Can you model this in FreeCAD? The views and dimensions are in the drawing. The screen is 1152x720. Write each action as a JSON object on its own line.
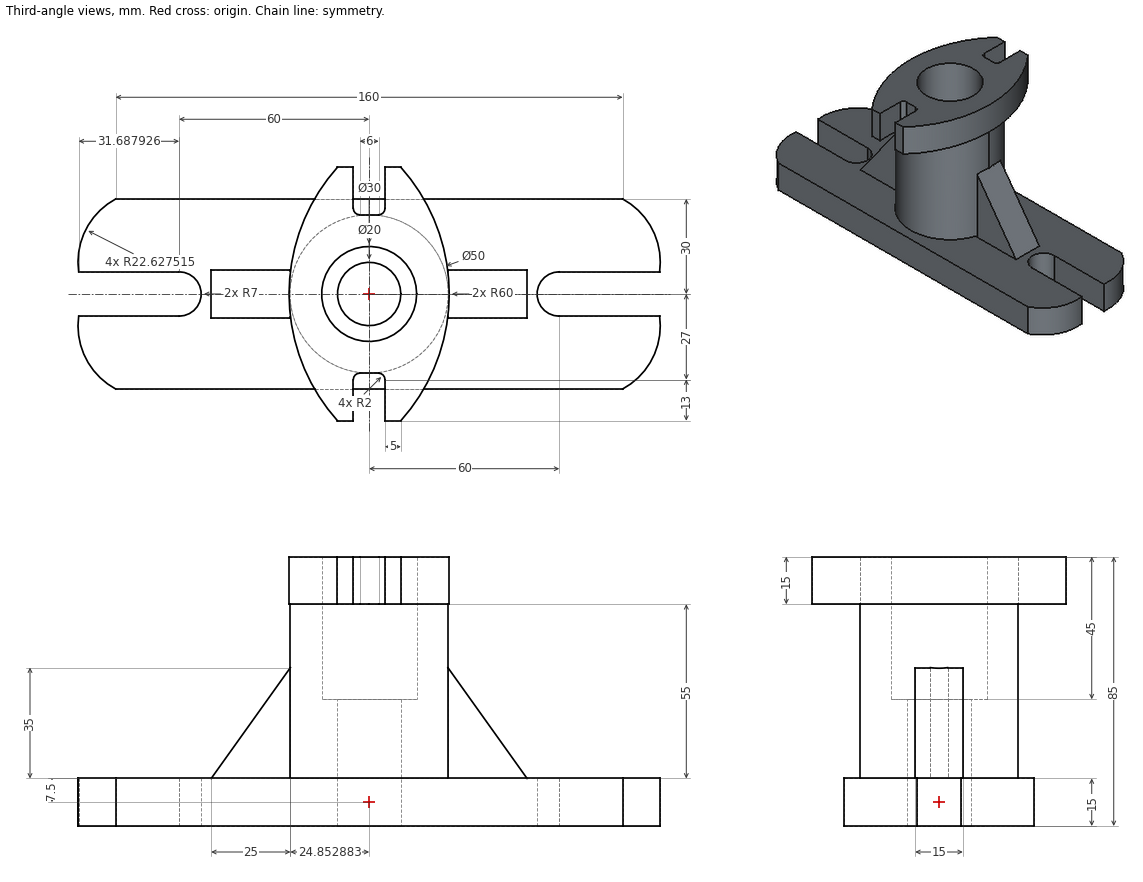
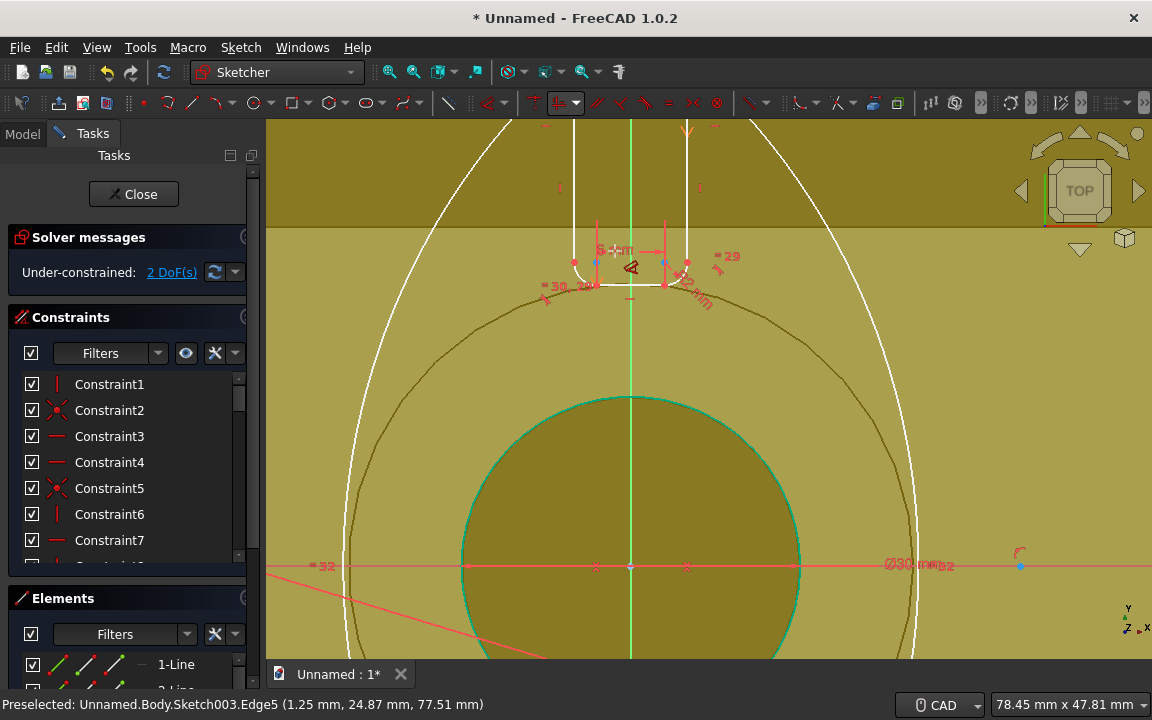
{"action": "scroll", "coordinate": [646, 286], "scroll_direction": "down", "scroll_amount": 5}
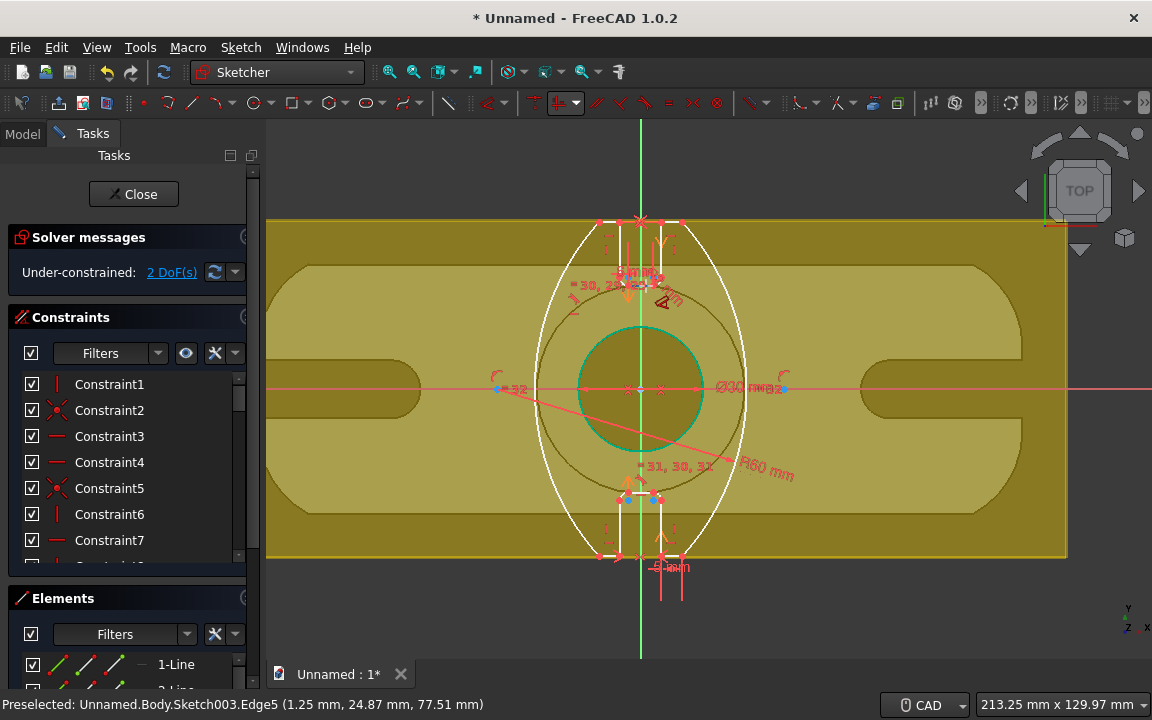
{"action": "left_click", "coordinate": [661, 518]}
{"action": "left_click", "coordinate": [695, 516]}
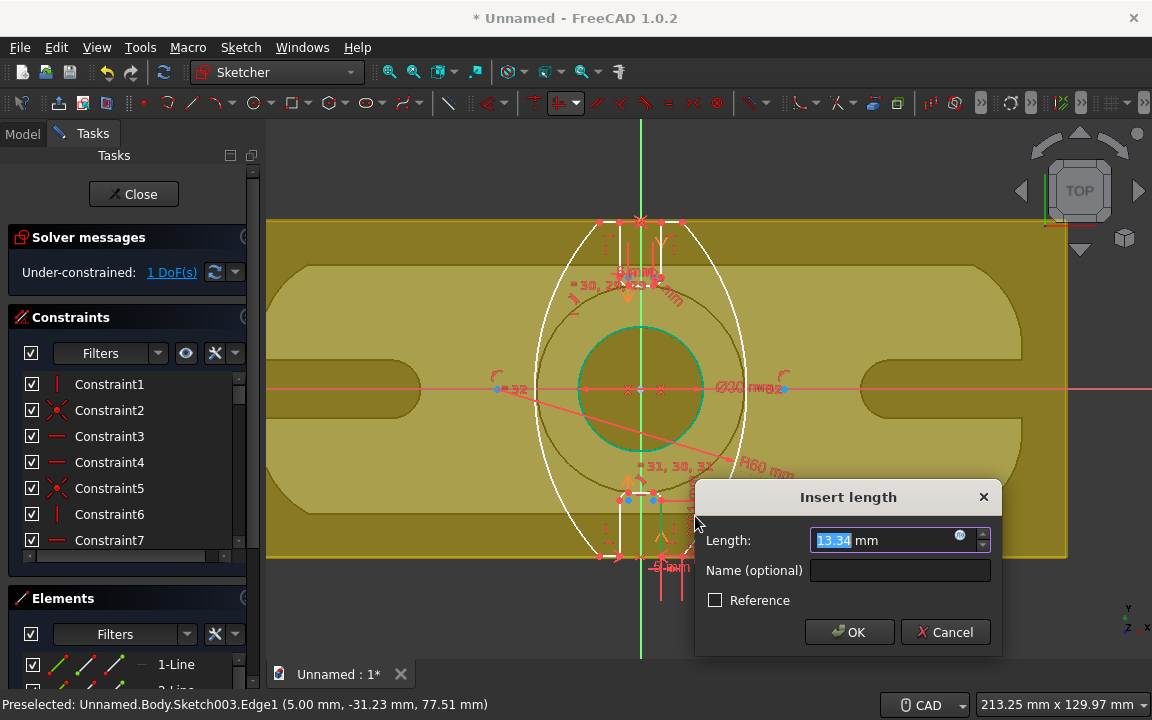
{"action": "type", "text": "13"}
{"action": "key", "text": "Return"}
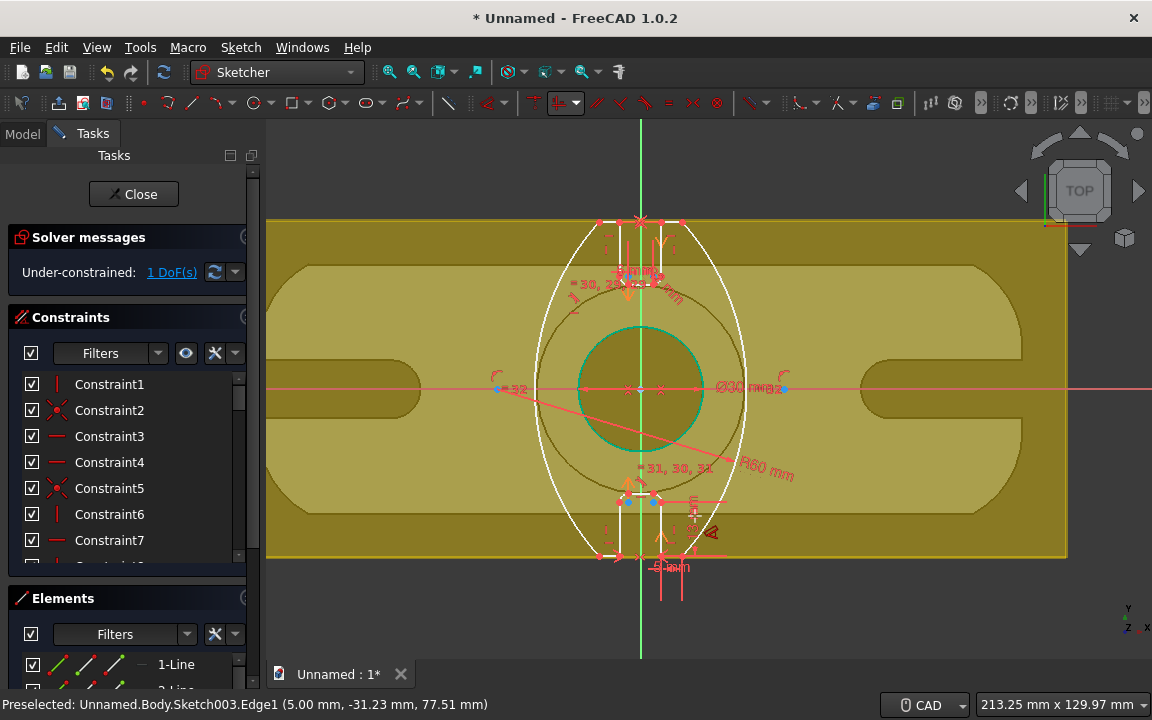
{"action": "scroll", "coordinate": [661, 502], "scroll_direction": "up", "scroll_amount": 2}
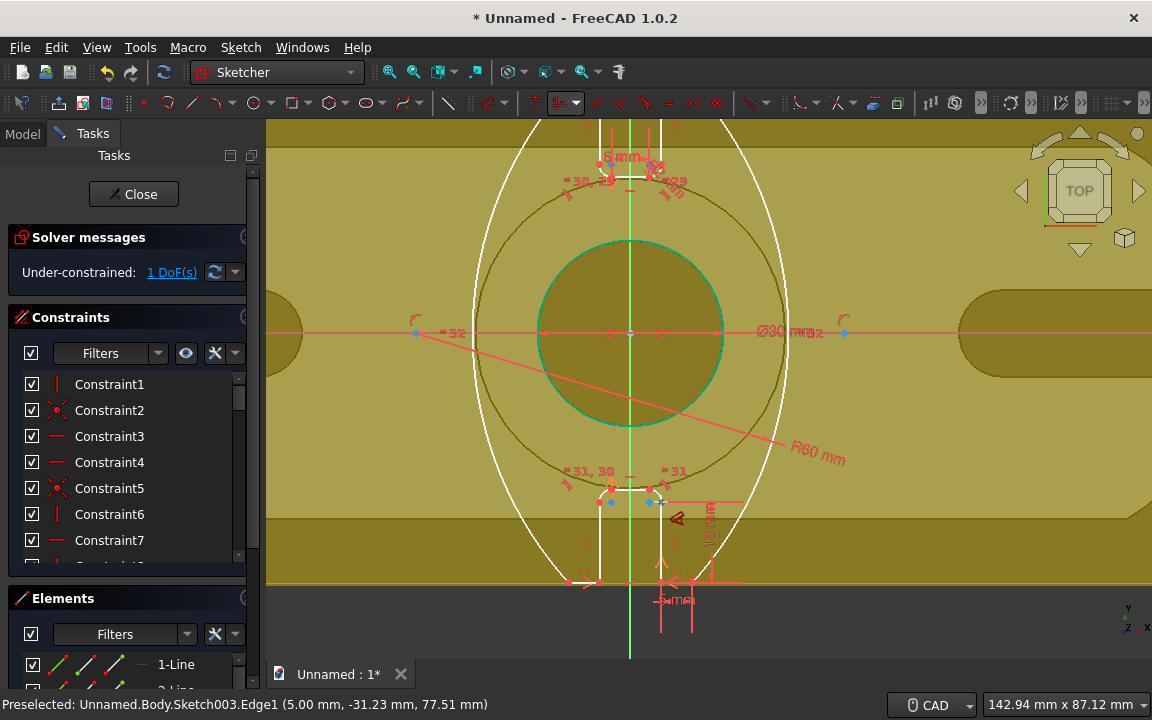
{"action": "left_click", "coordinate": [661, 502]}
{"action": "left_click", "coordinate": [695, 418]}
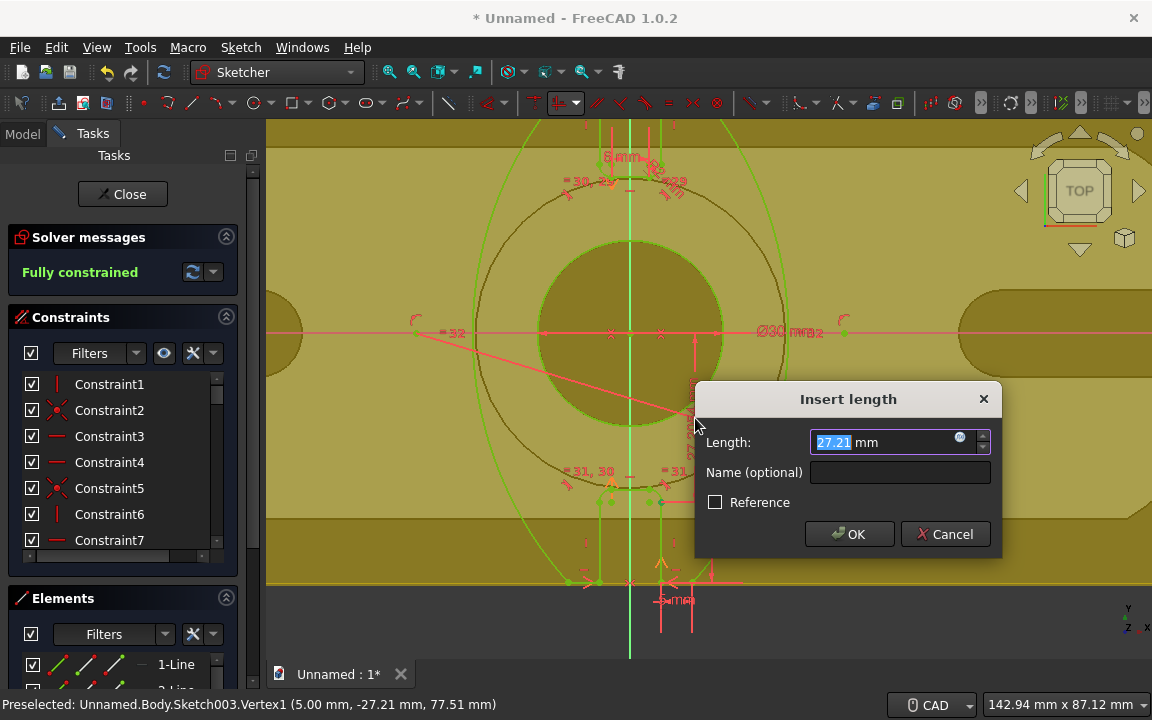
{"action": "type", "text": "27"}
{"action": "key", "text": "Return"}
{"action": "key", "text": "Escape"}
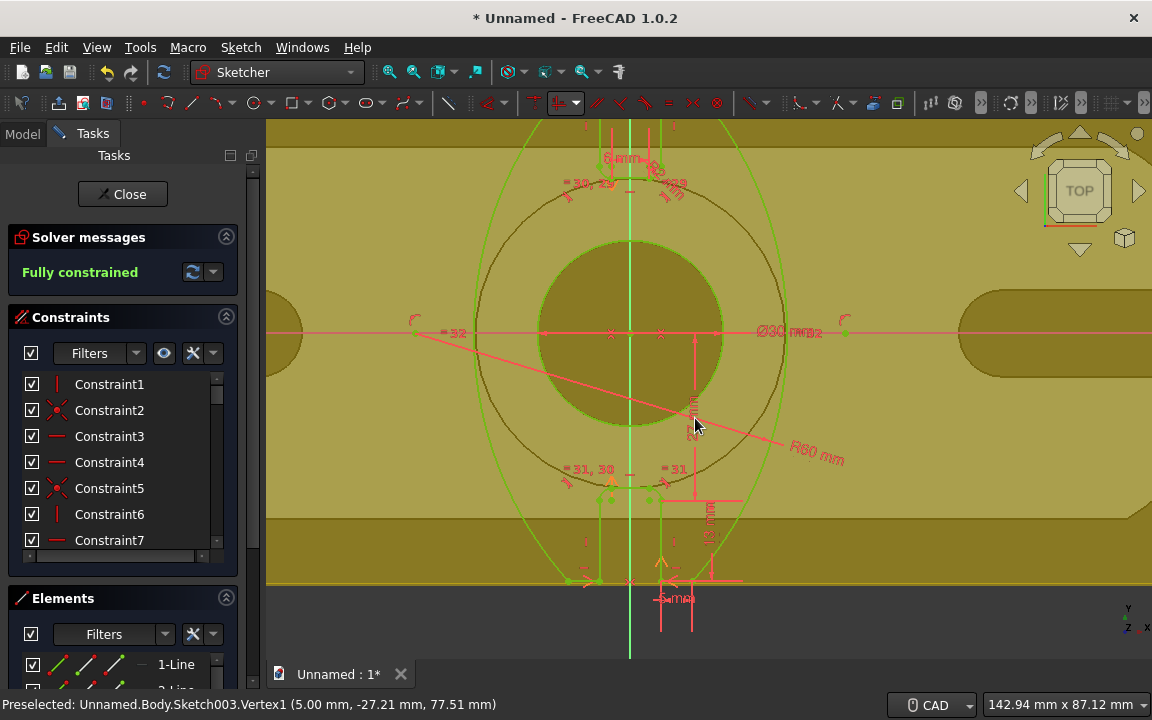
{"action": "left_click", "coordinate": [123, 194]}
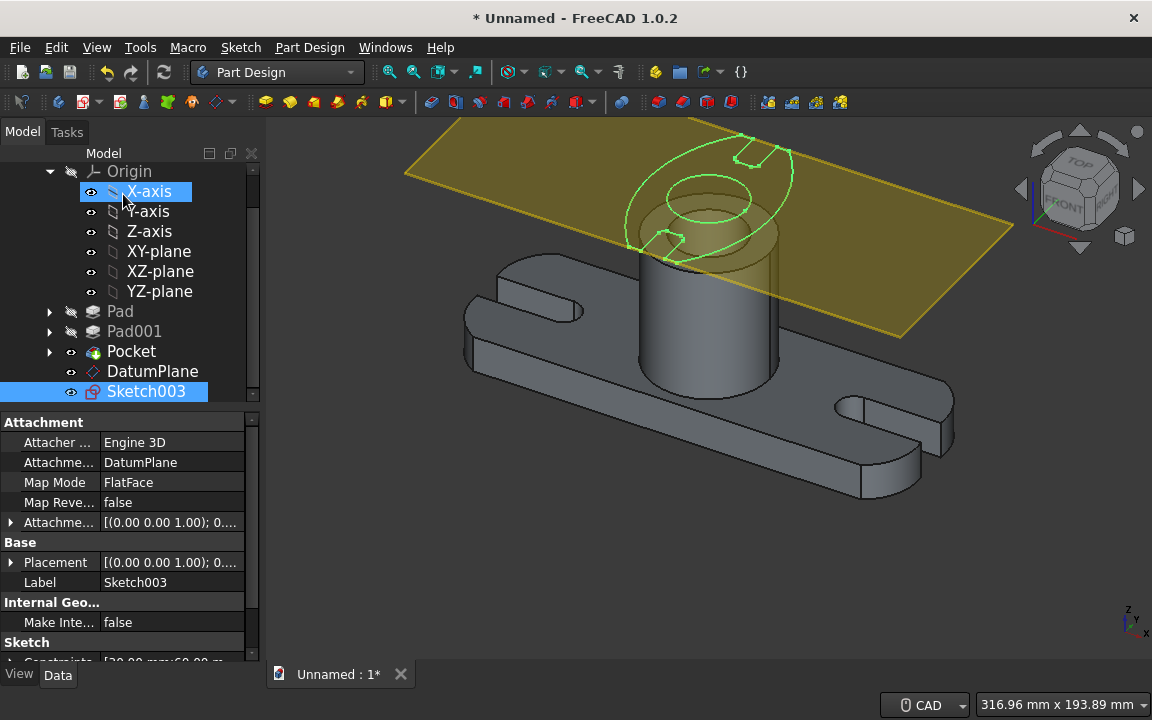
{"action": "left_click", "coordinate": [266, 102]}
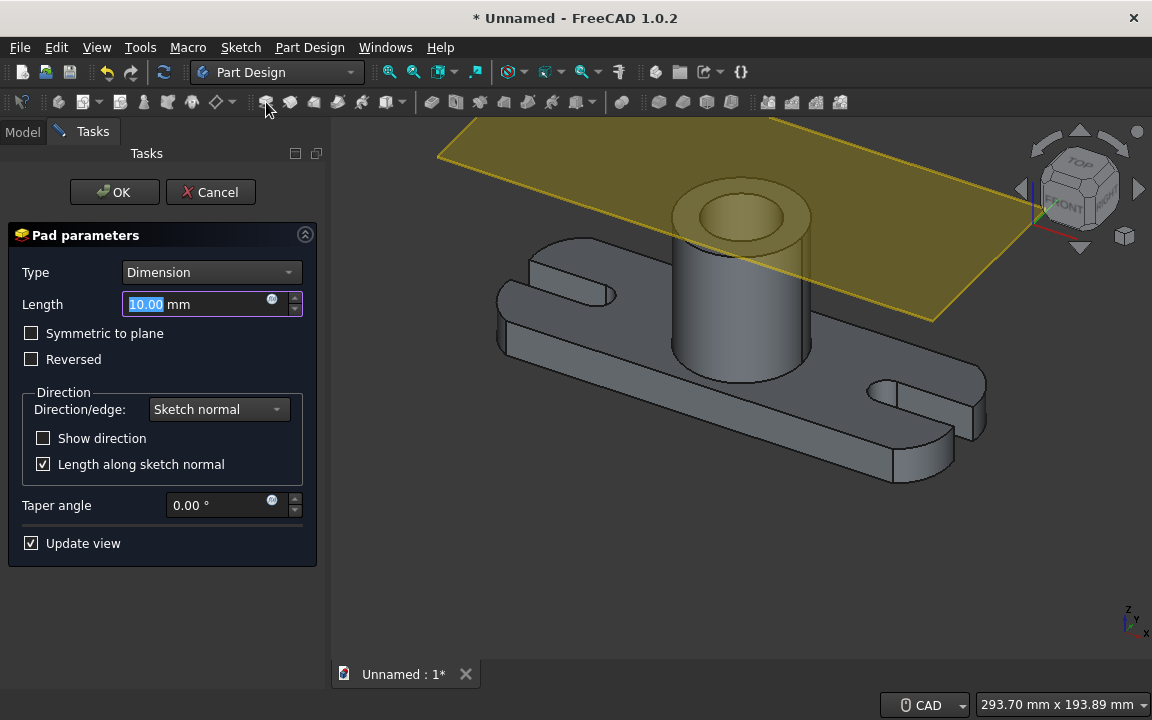
{"action": "type", "text": "15"}
{"action": "key", "text": "Tab"}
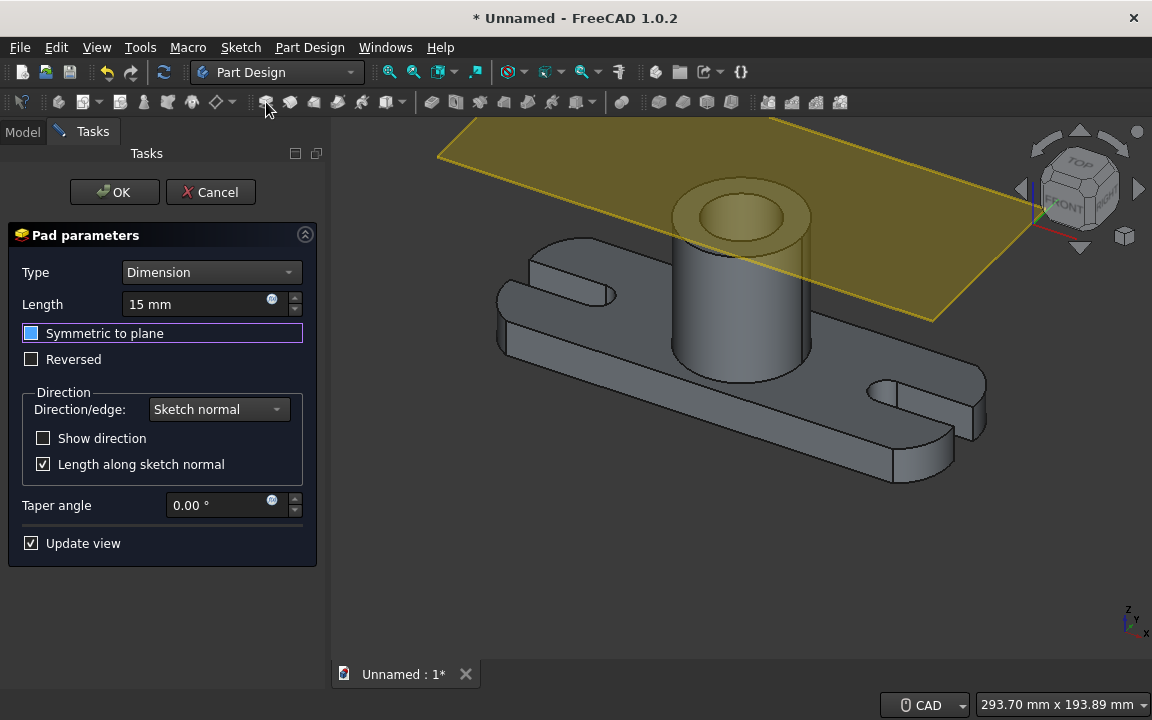
{"action": "left_click", "coordinate": [30, 359]}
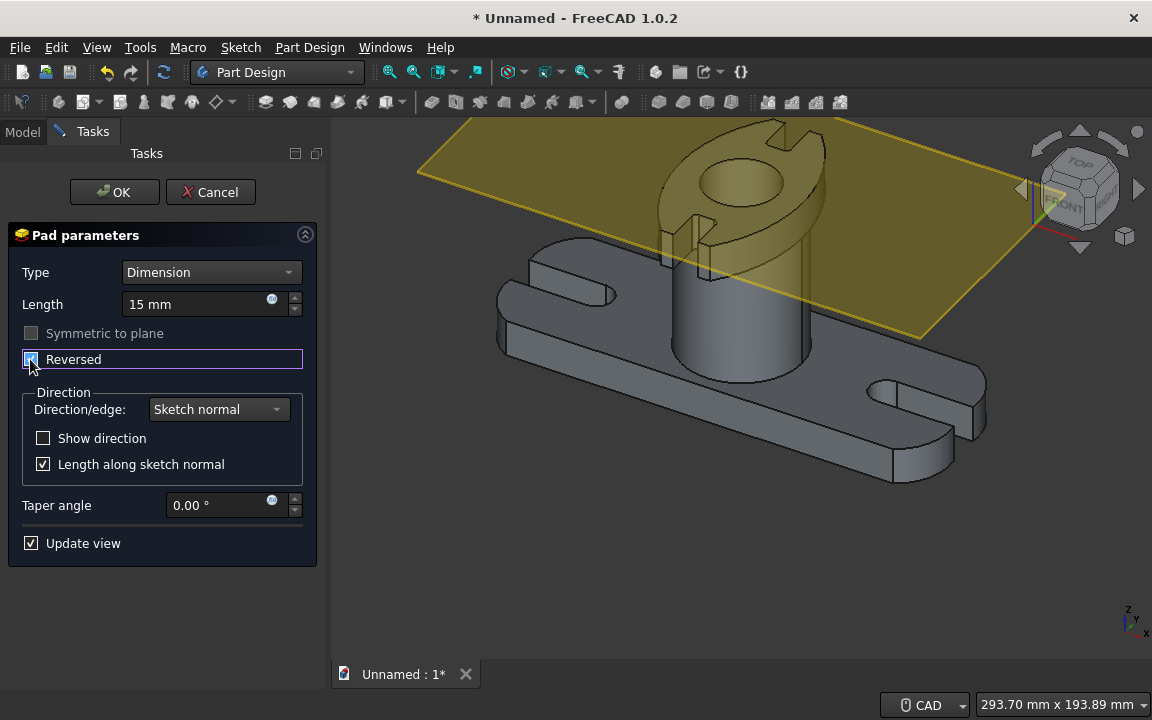
{"action": "left_click", "coordinate": [115, 192]}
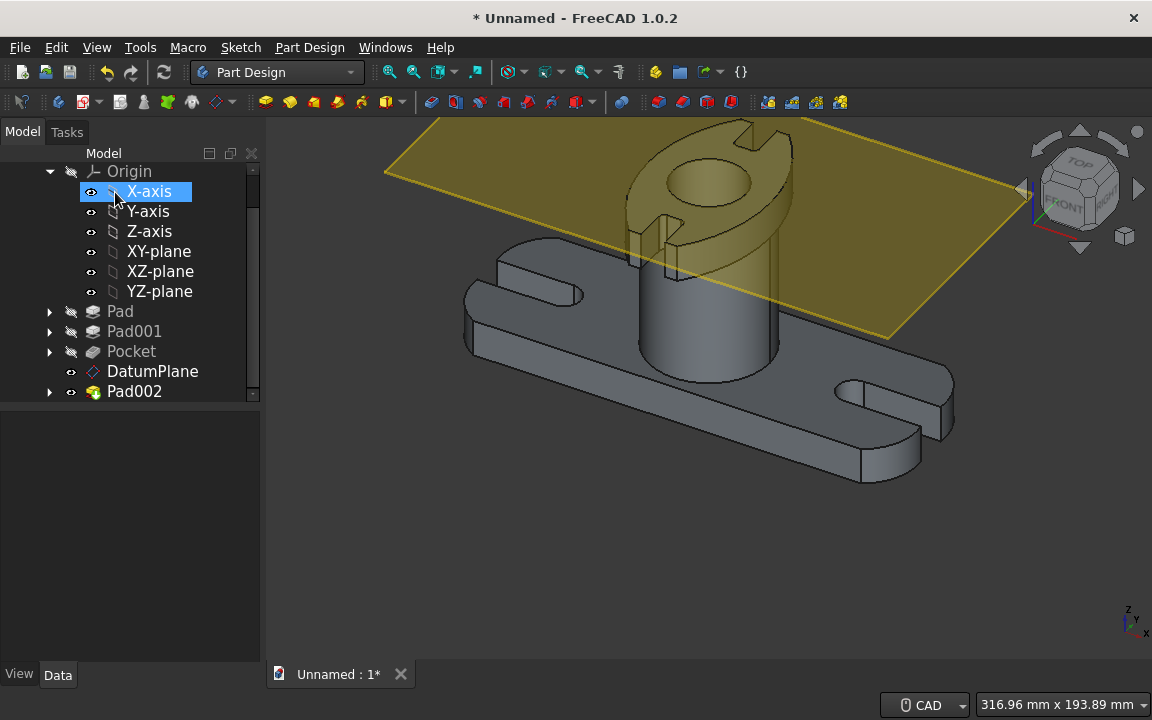
{"action": "left_click", "coordinate": [116, 372]}
{"action": "key", "text": "space"}